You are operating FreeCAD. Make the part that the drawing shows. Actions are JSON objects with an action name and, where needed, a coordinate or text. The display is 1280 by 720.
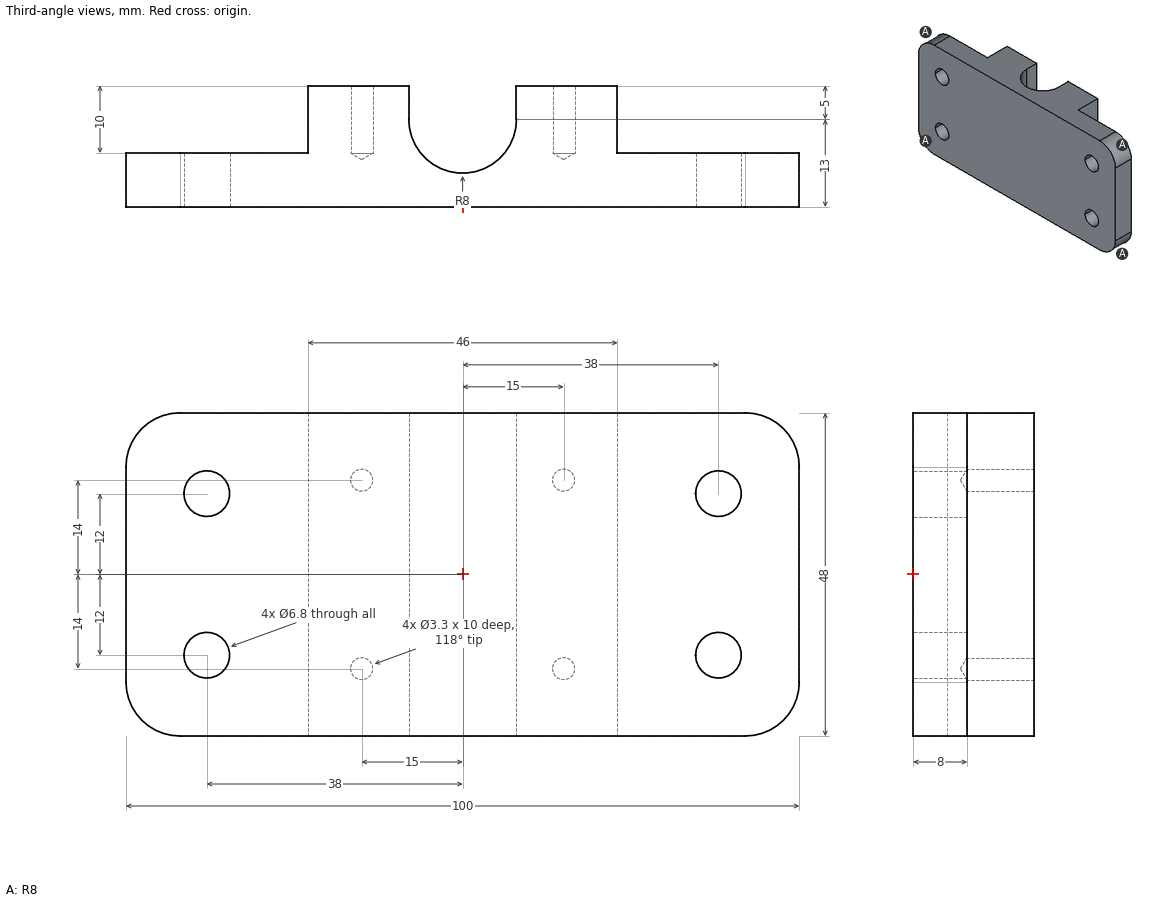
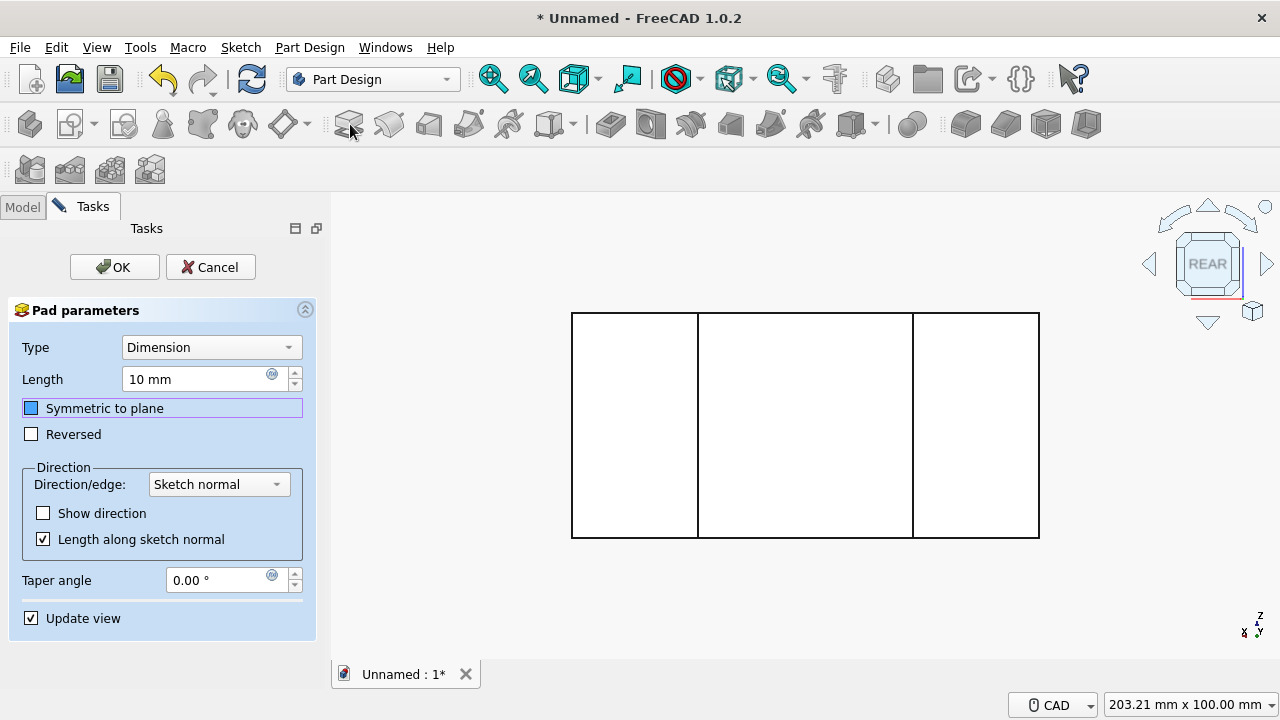
{"action": "left_click", "coordinate": [115, 267]}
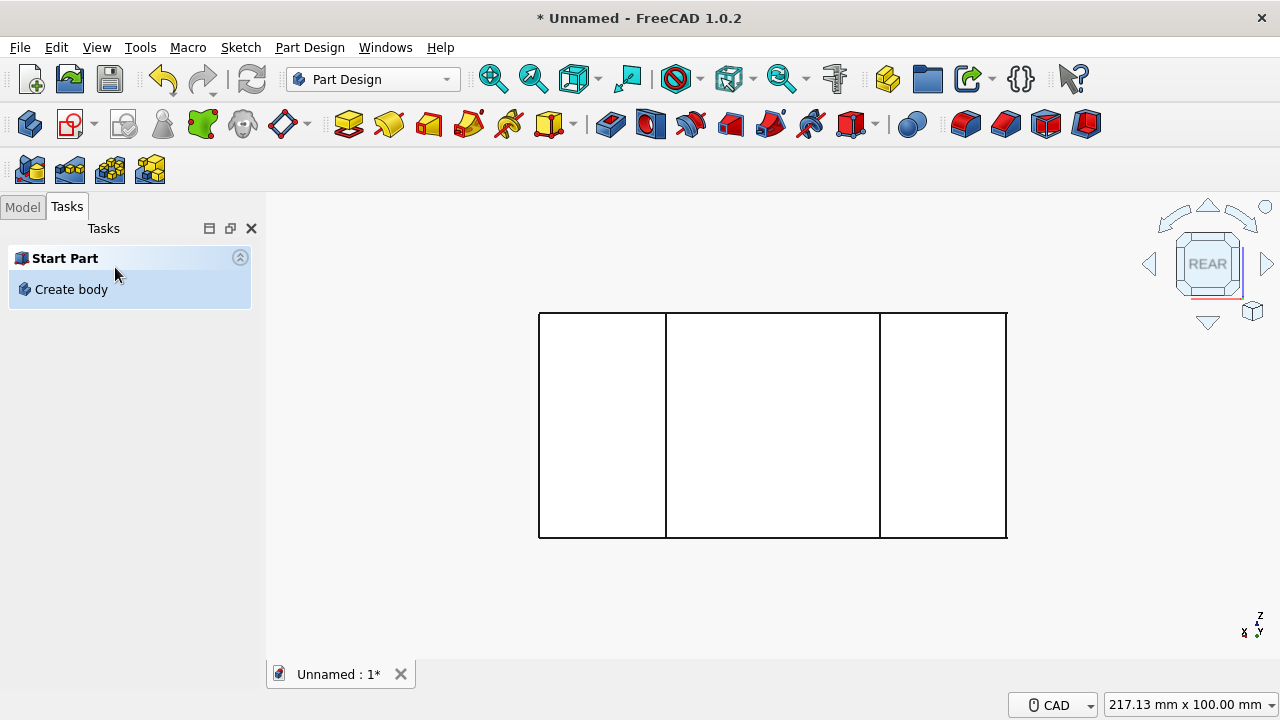
{"action": "key", "text": "0"}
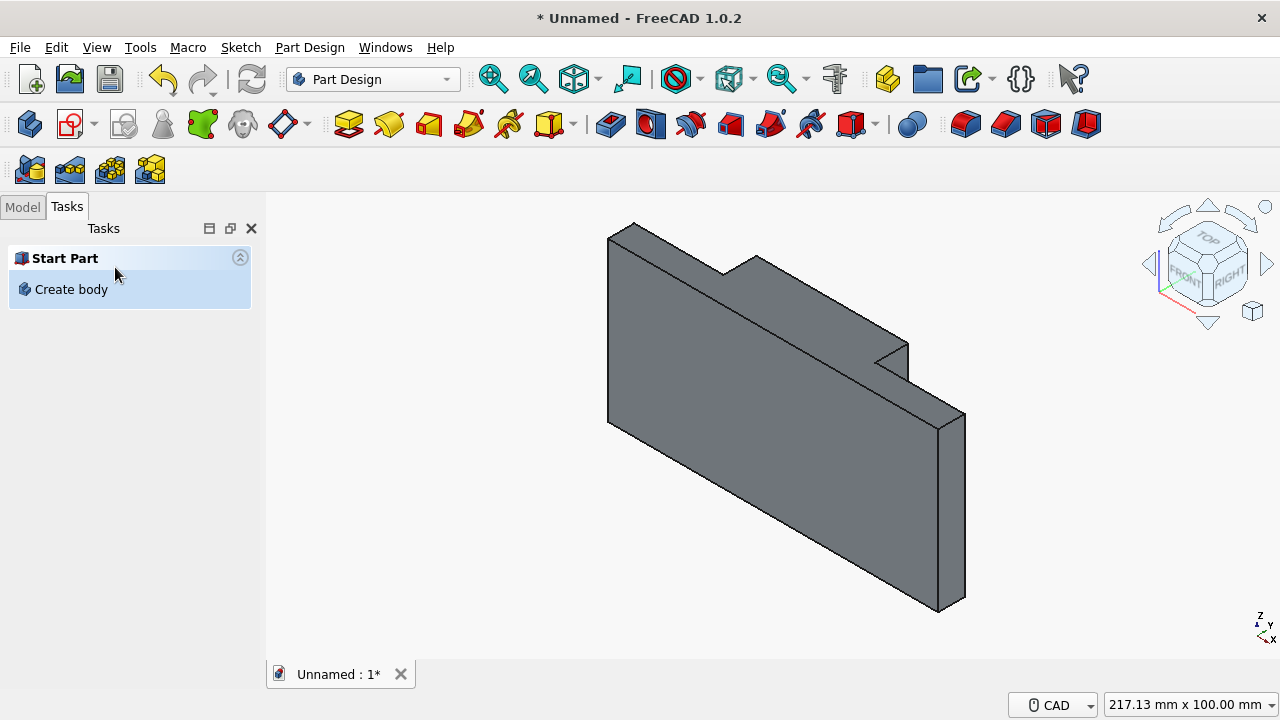
{"action": "left_click", "coordinate": [803, 316]}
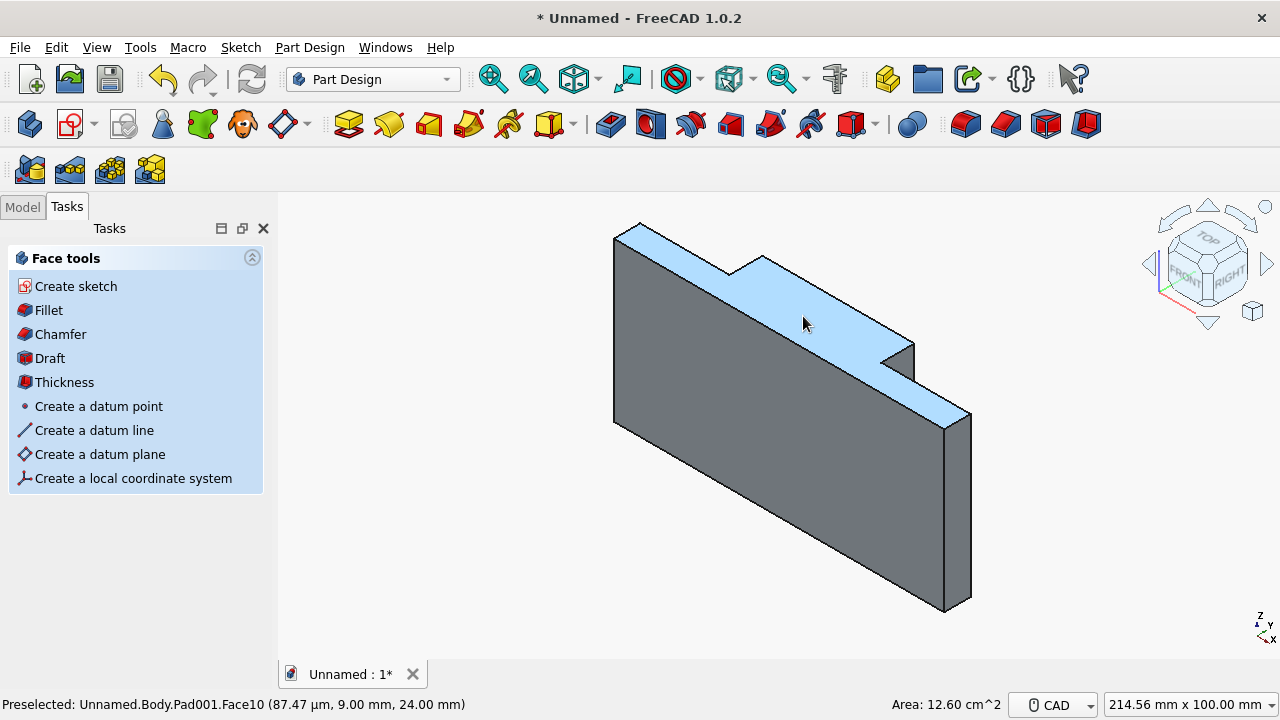
{"action": "left_click", "coordinate": [70, 124]}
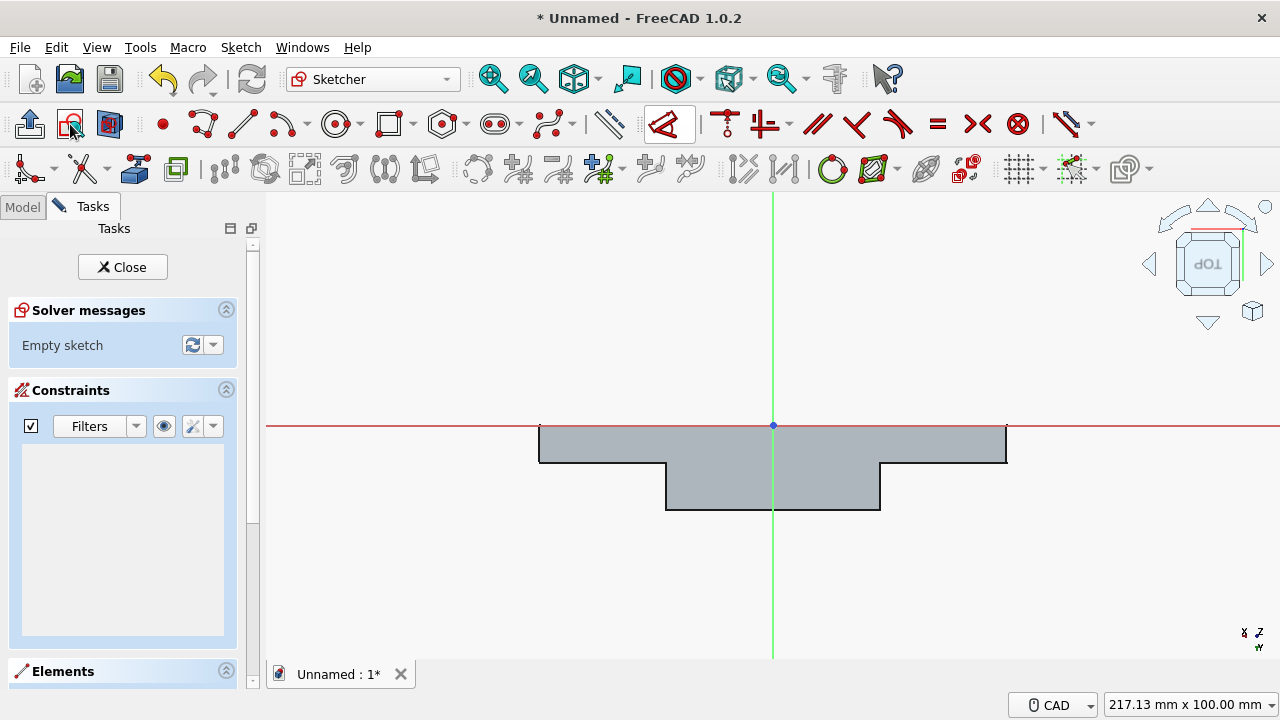
{"action": "scroll", "coordinate": [803, 486], "scroll_direction": "up", "scroll_amount": 6}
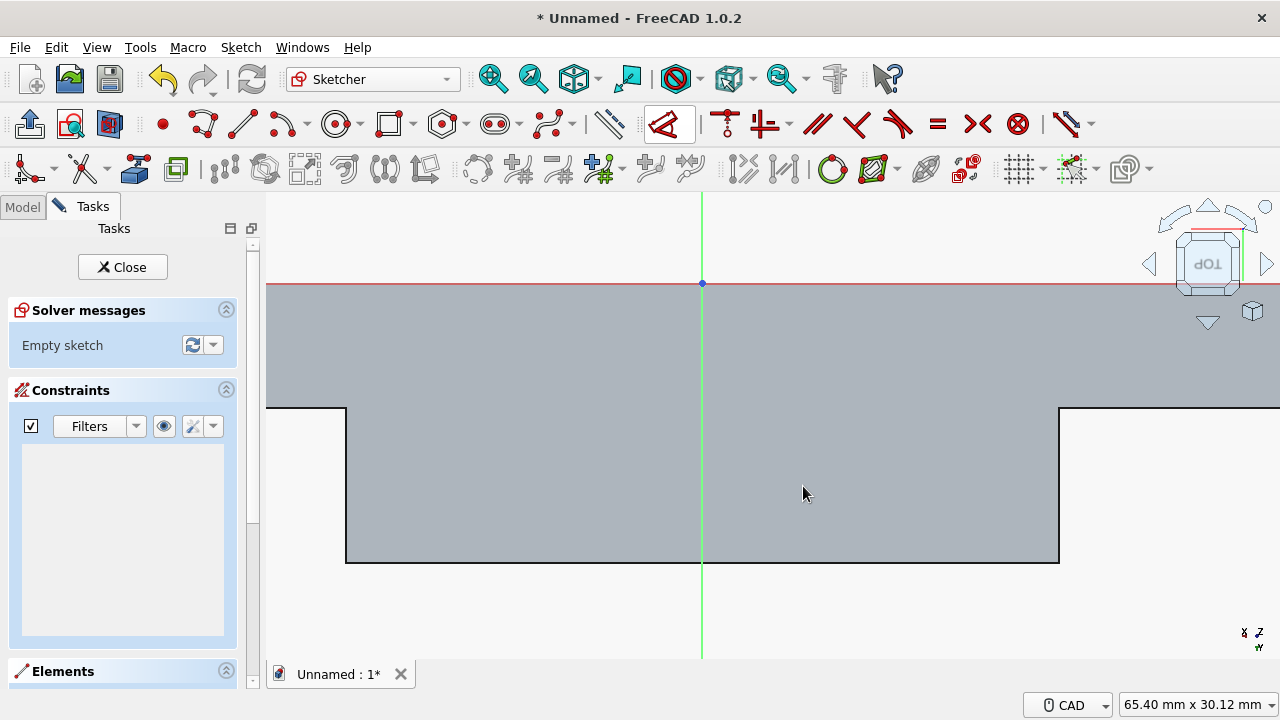
{"action": "left_click", "coordinate": [204, 124]}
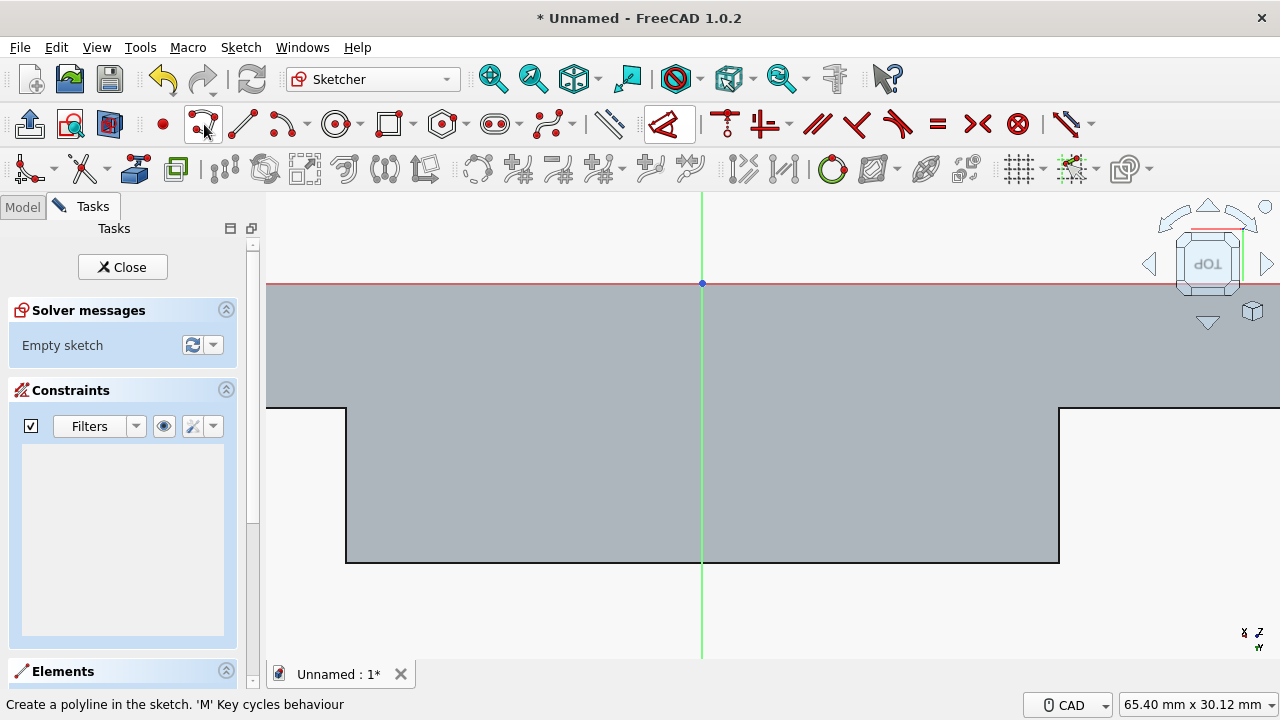
{"action": "left_click", "coordinate": [578, 485]}
{"action": "left_click", "coordinate": [578, 563]}
{"action": "left_click", "coordinate": [826, 563]}
{"action": "left_click", "coordinate": [826, 485]}
{"action": "right_click", "coordinate": [826, 485]}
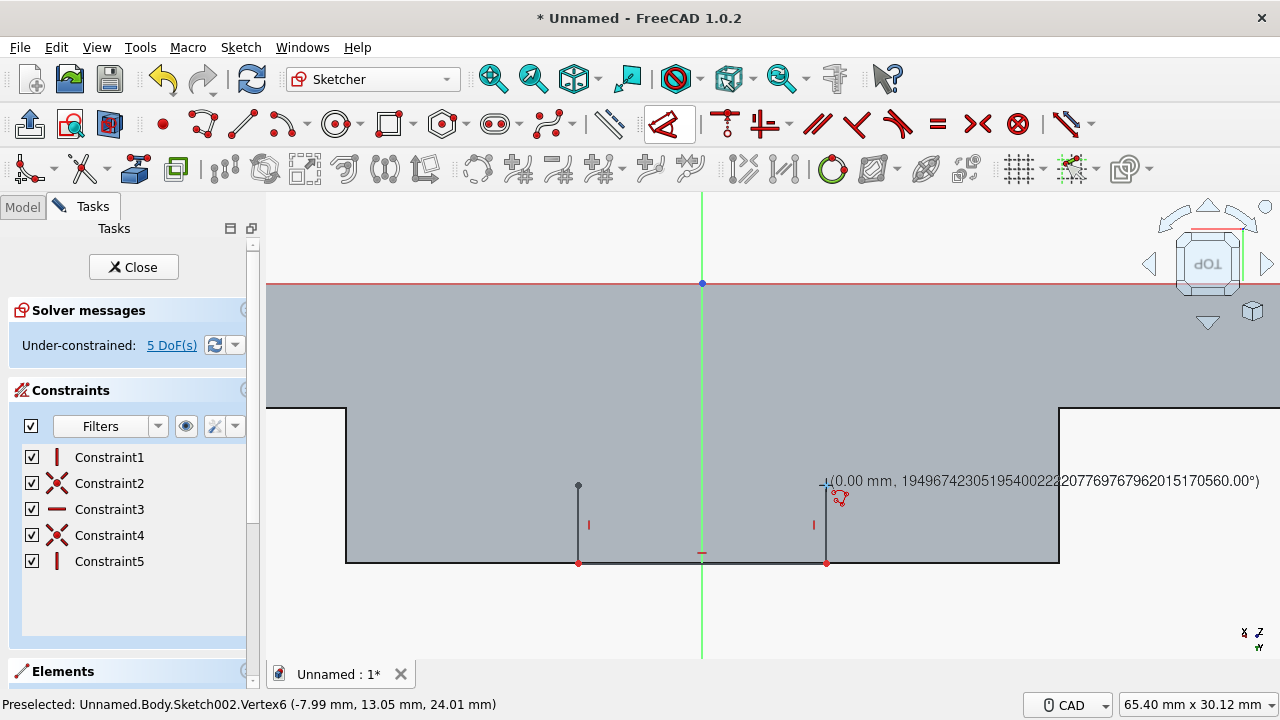
{"action": "left_click", "coordinate": [310, 124]}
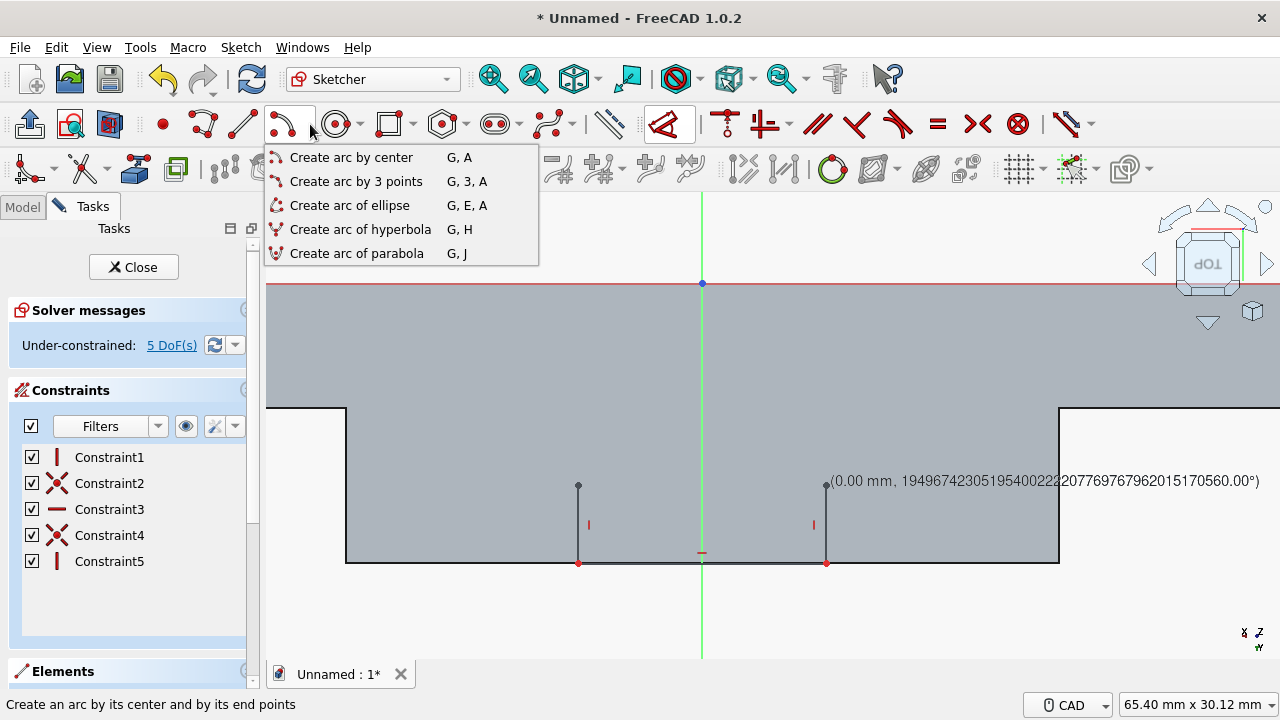
{"action": "left_click", "coordinate": [402, 181]}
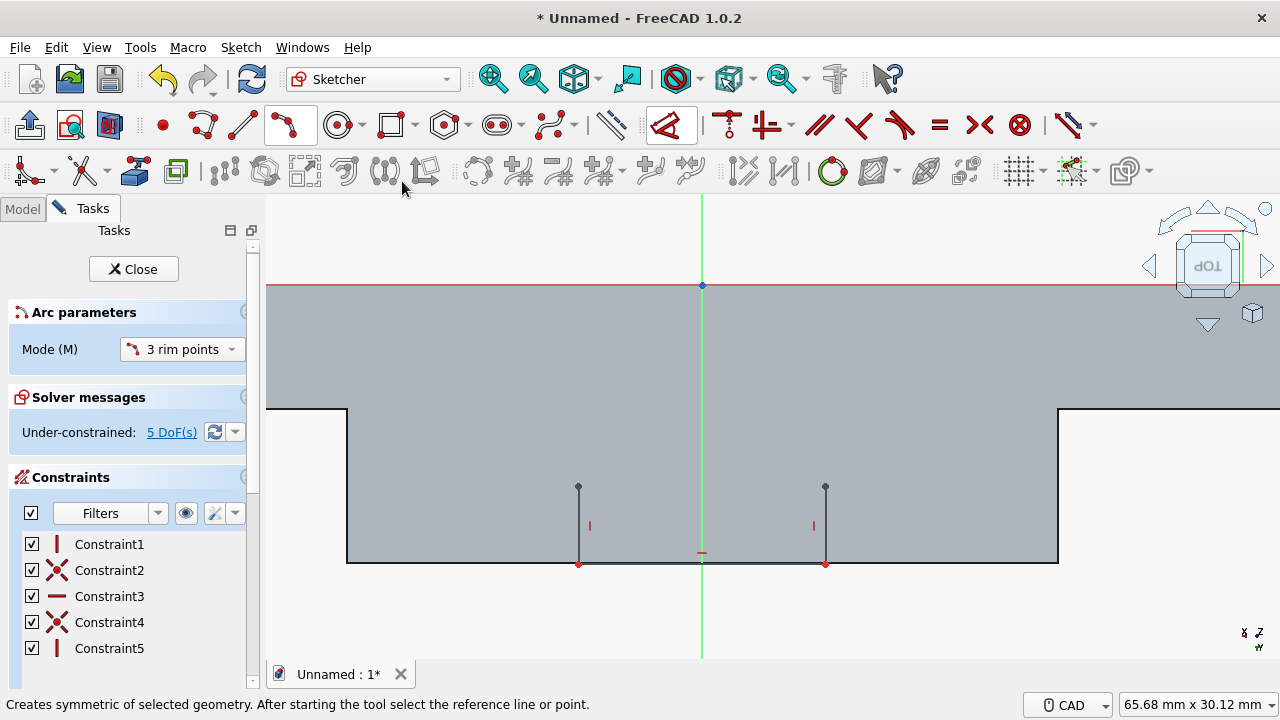
{"action": "left_click", "coordinate": [826, 487]}
{"action": "left_click", "coordinate": [579, 487]}
{"action": "left_click", "coordinate": [741, 369]}
{"action": "key", "text": "Escape"}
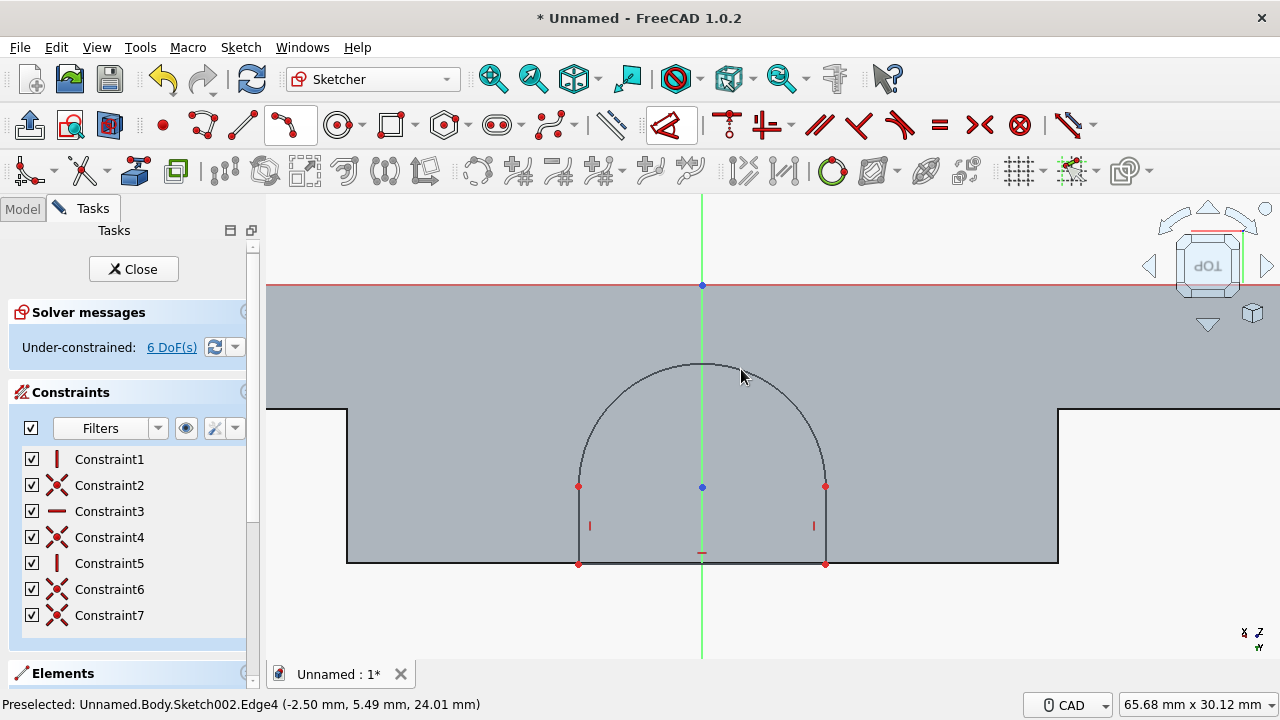
{"action": "left_click", "coordinate": [579, 510]}